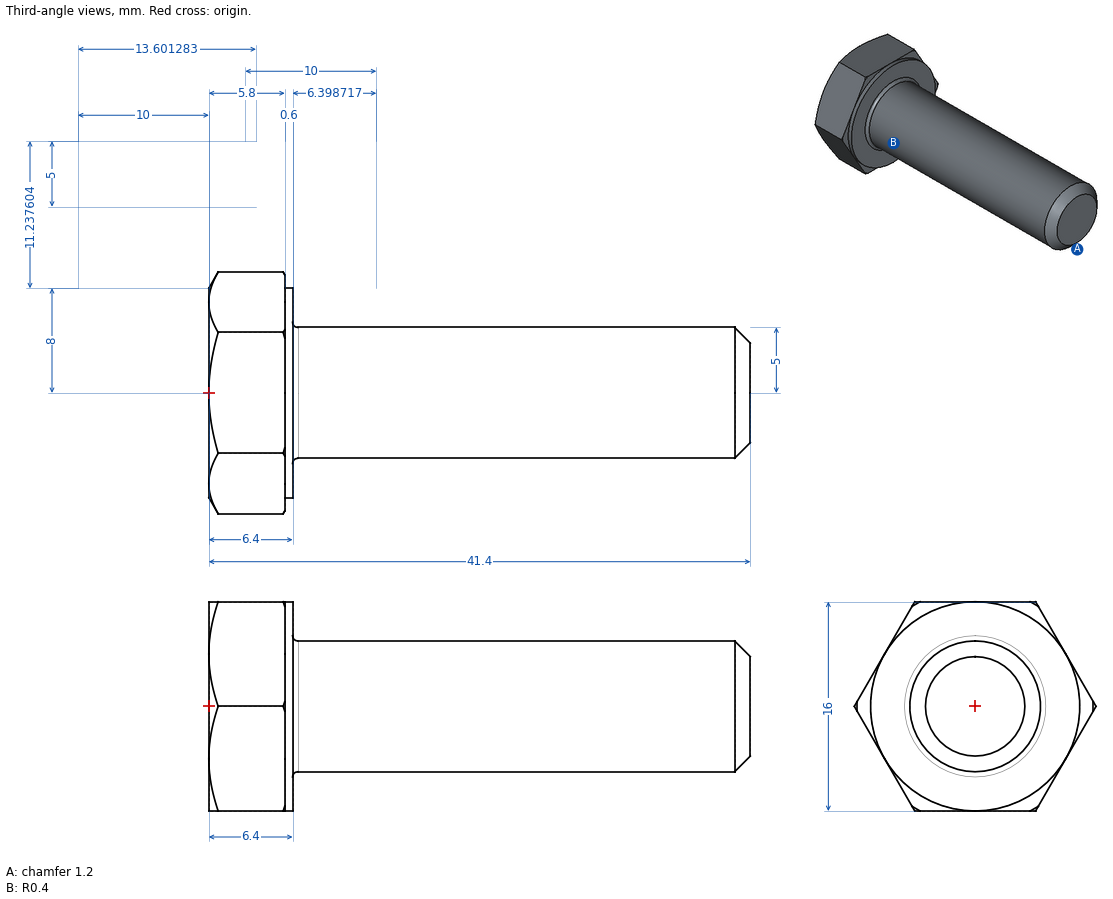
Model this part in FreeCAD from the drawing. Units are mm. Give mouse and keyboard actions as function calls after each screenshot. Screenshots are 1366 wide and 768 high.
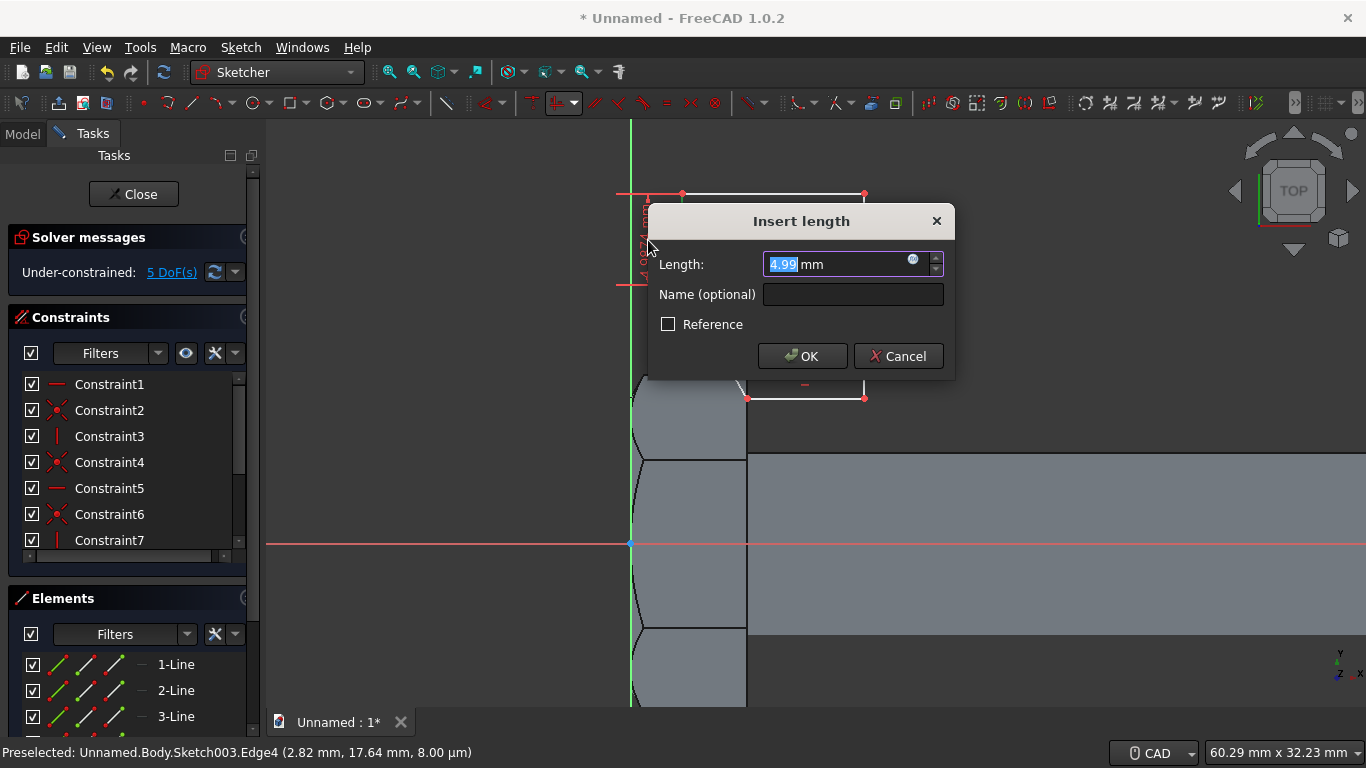
text(5)
key(Return)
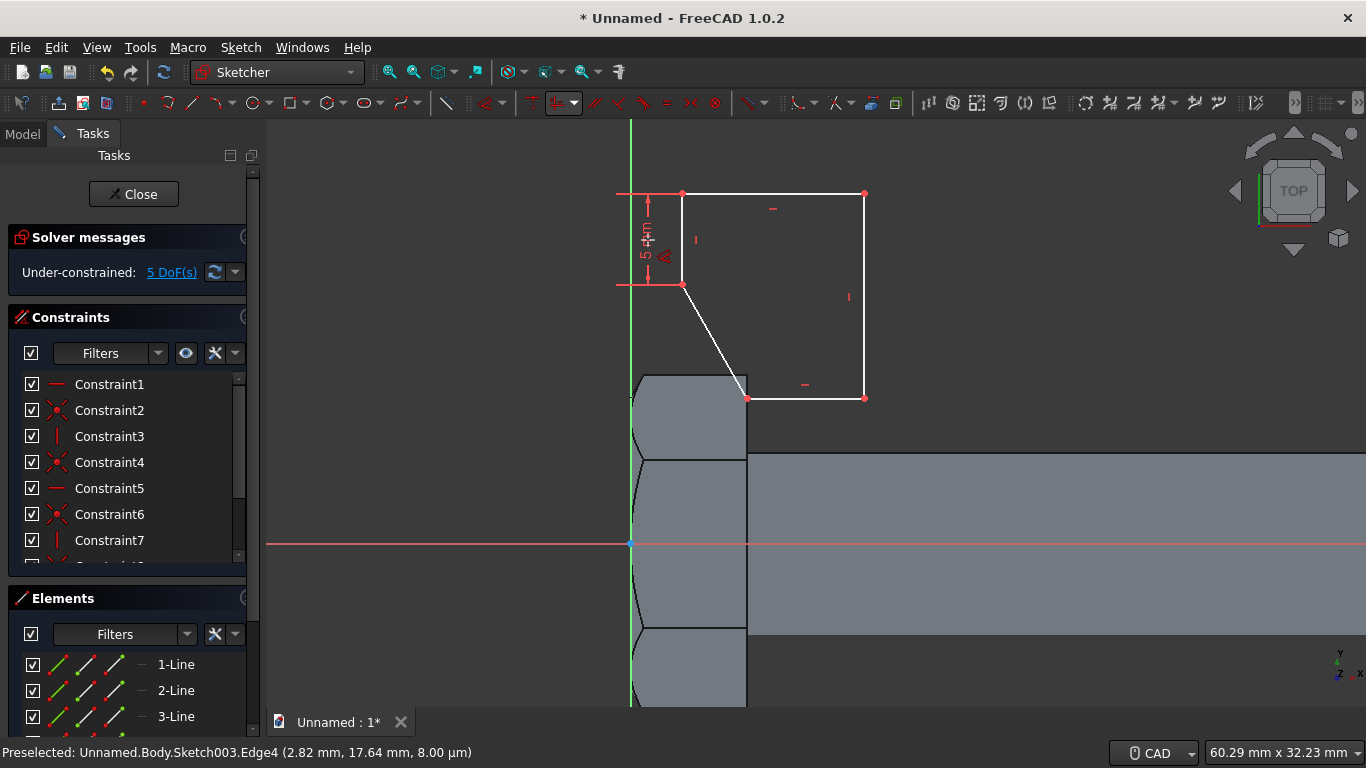
click(809, 194)
click(773, 160)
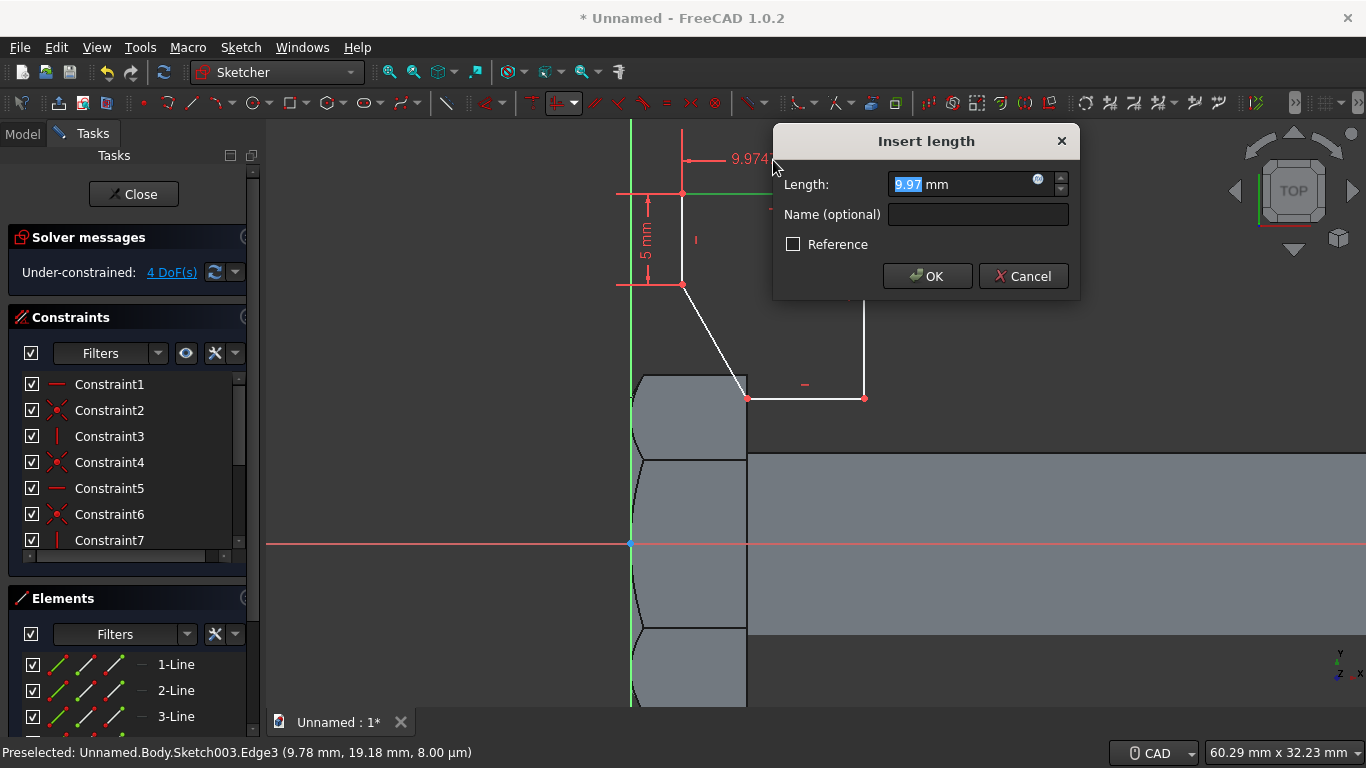
text(10)
key(Return)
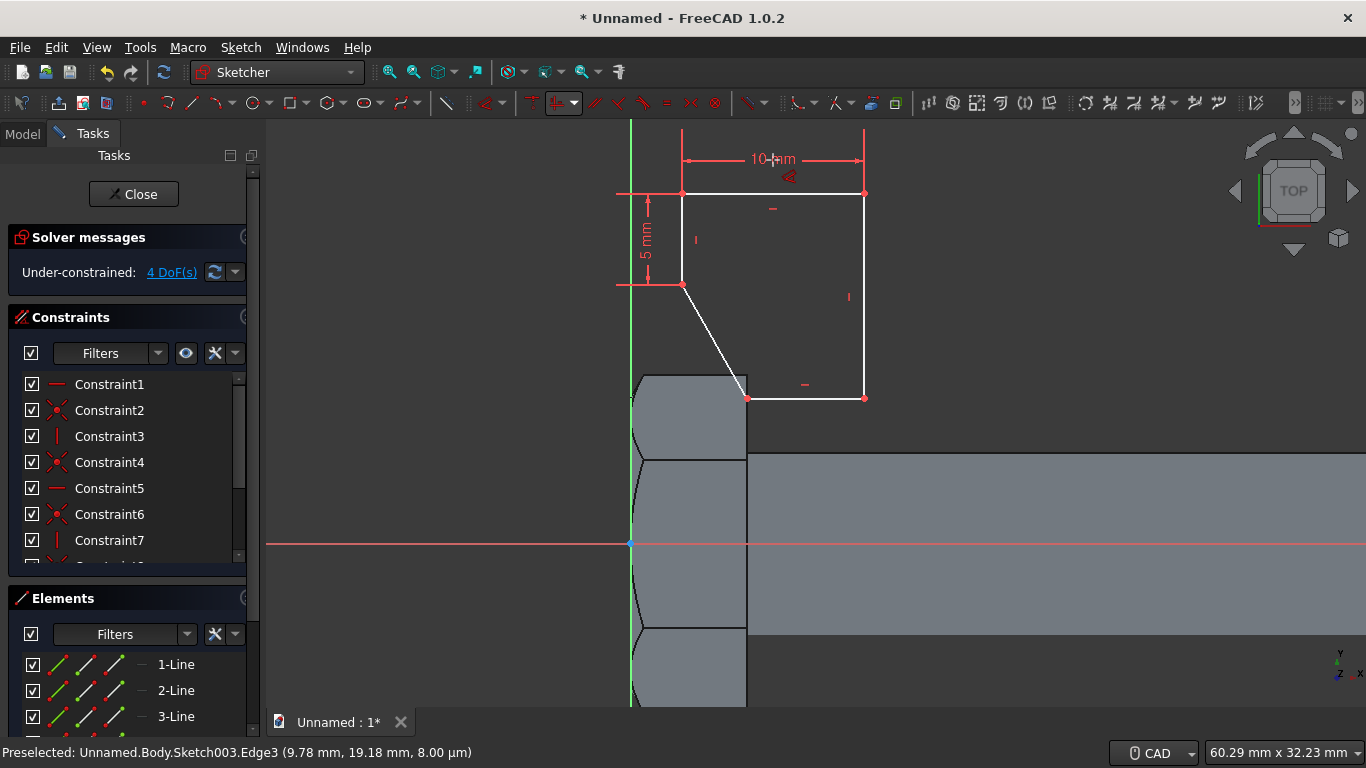
click(747, 399)
click(597, 471)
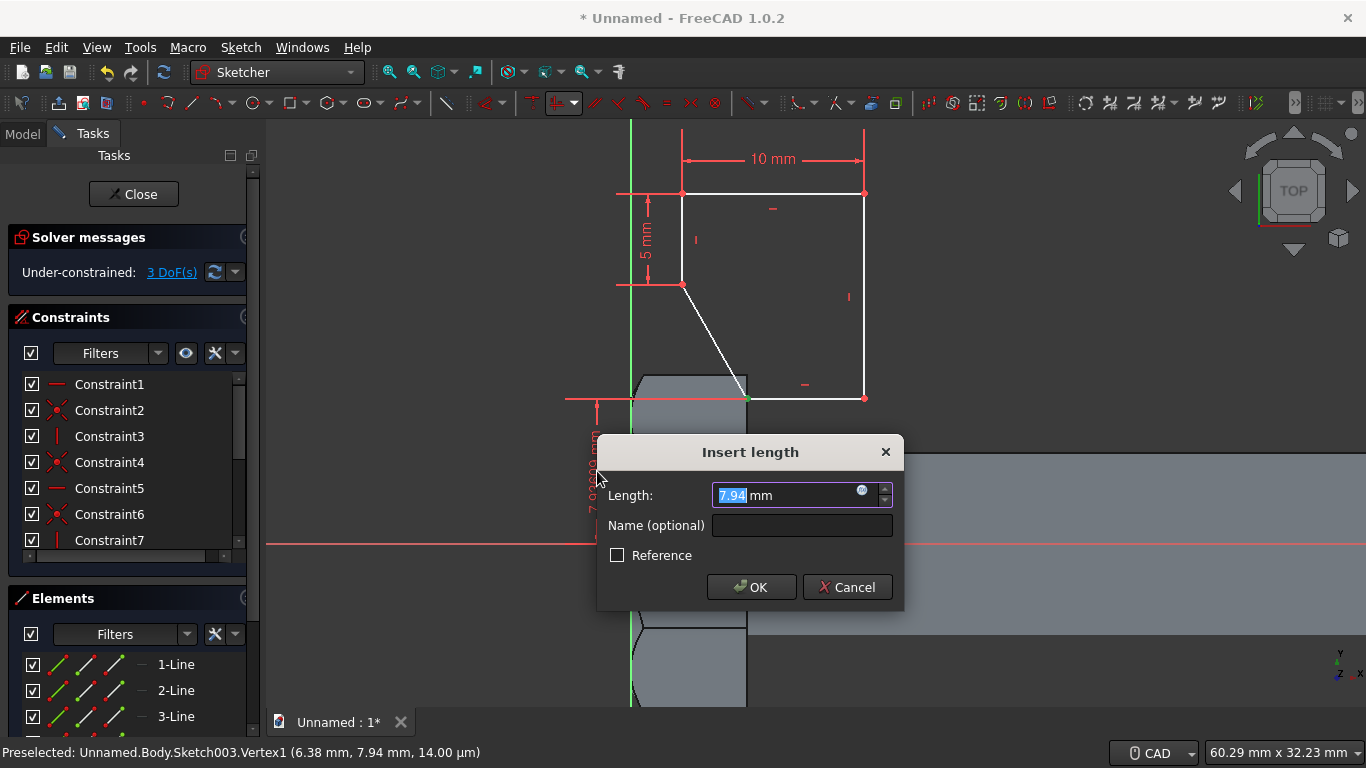
text(8)
key(Return)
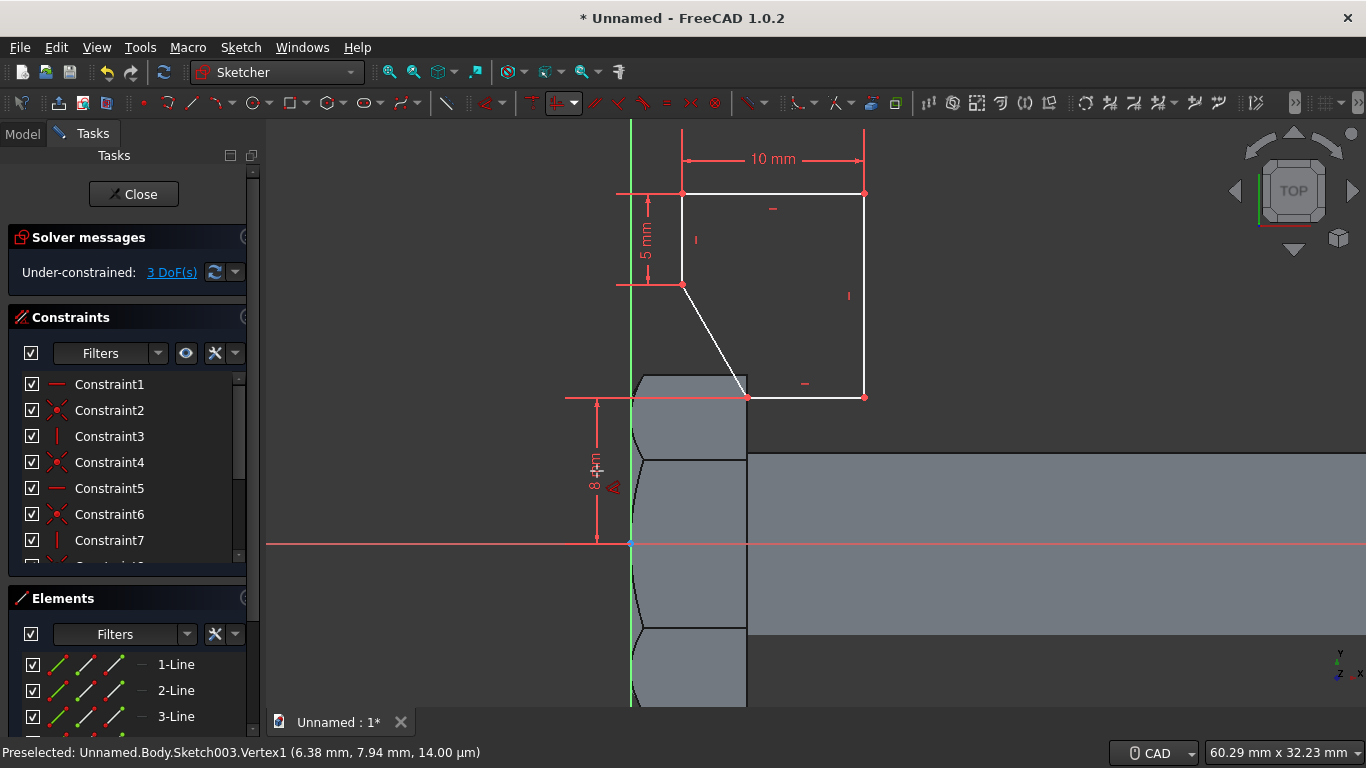
click(747, 398)
click(689, 578)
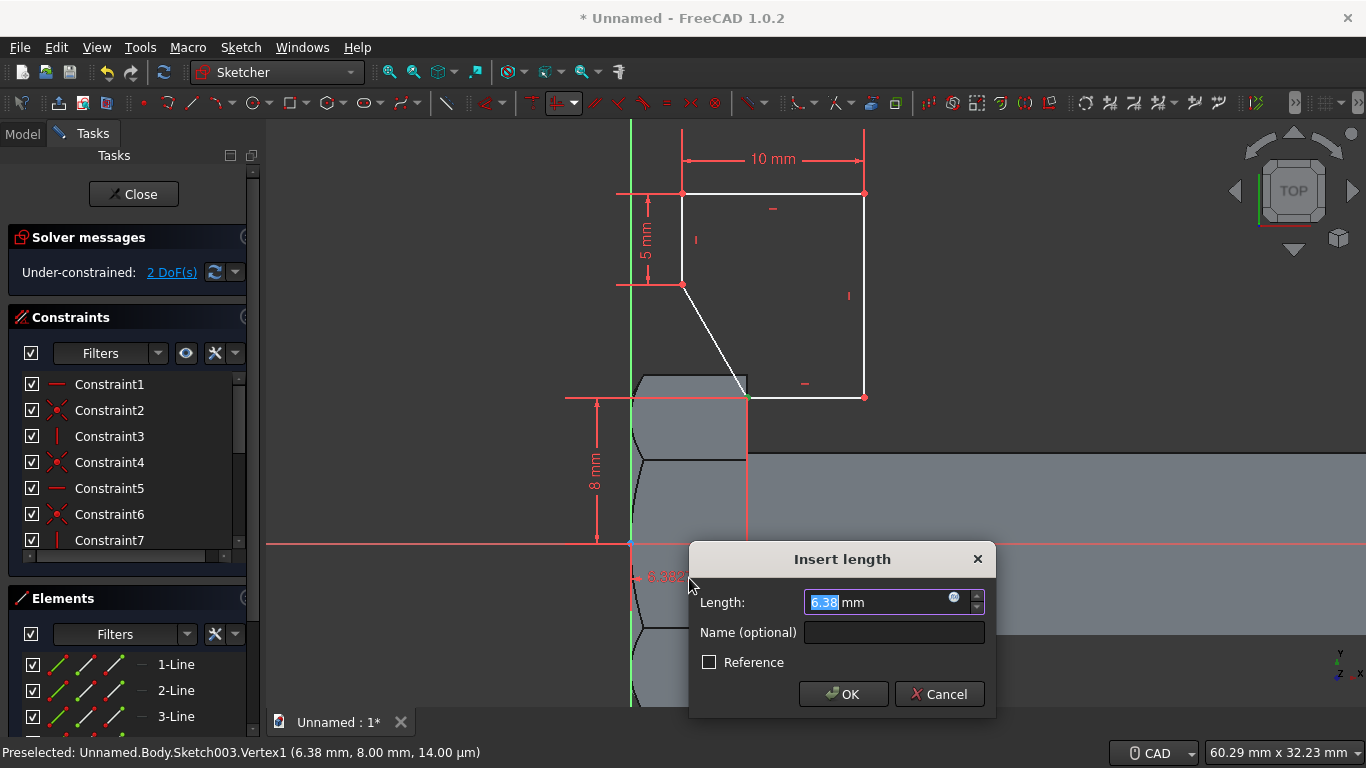
text(6.4)
key(Return)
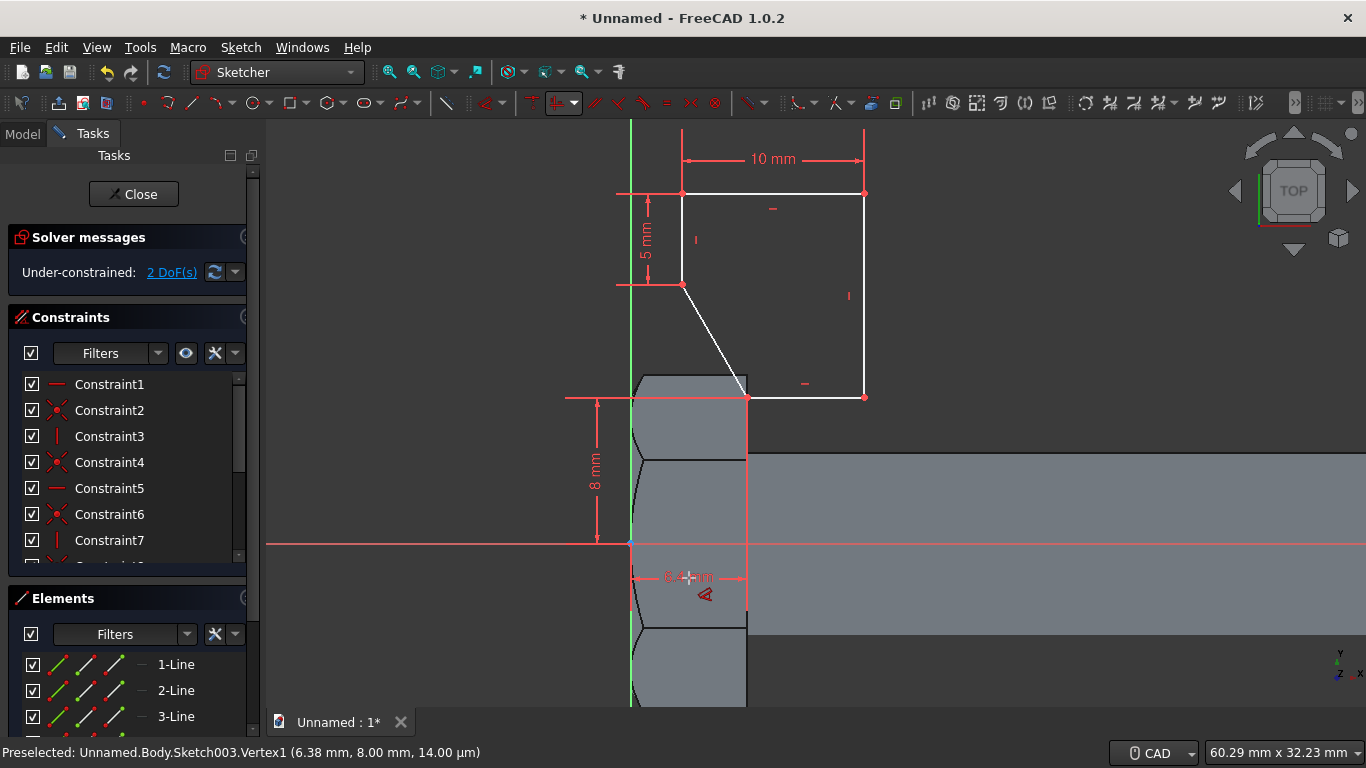
click(782, 398)
click(806, 432)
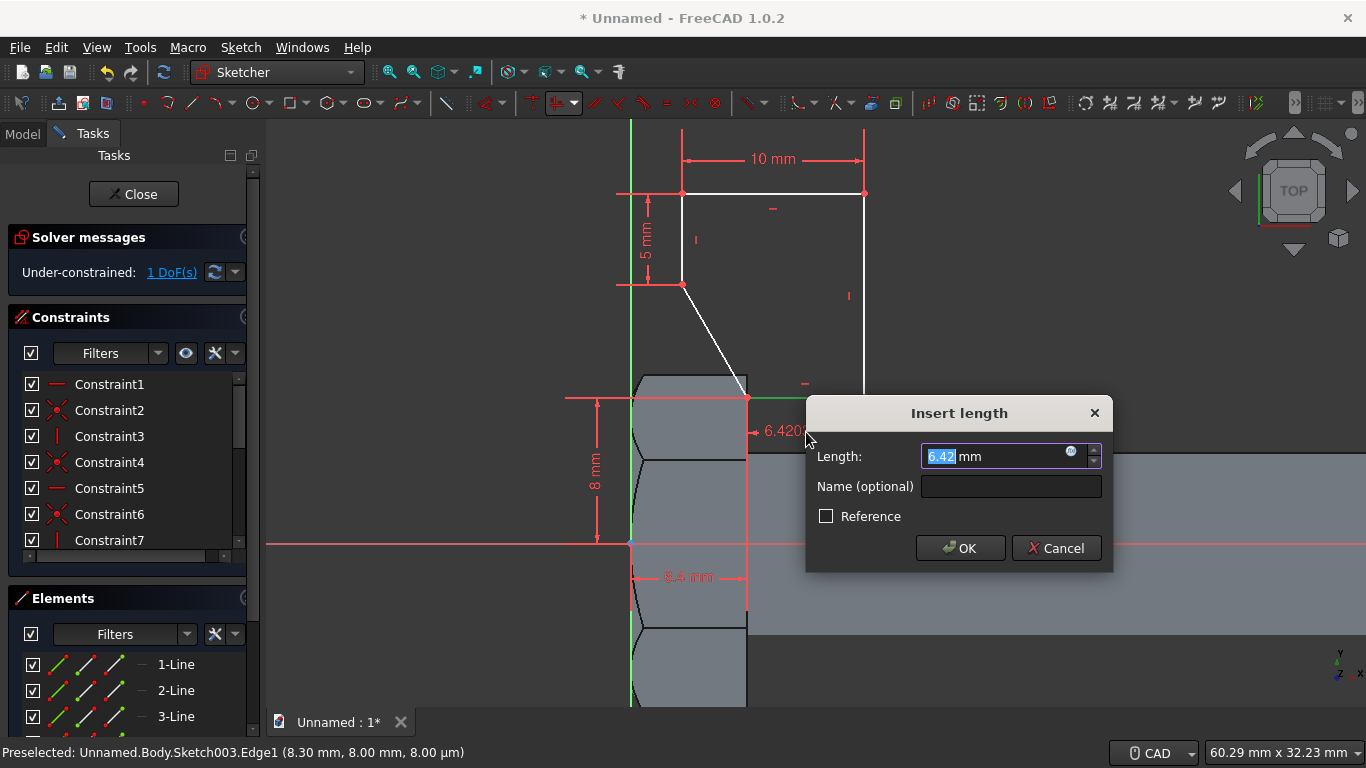
text(6.398717)
key(Return)